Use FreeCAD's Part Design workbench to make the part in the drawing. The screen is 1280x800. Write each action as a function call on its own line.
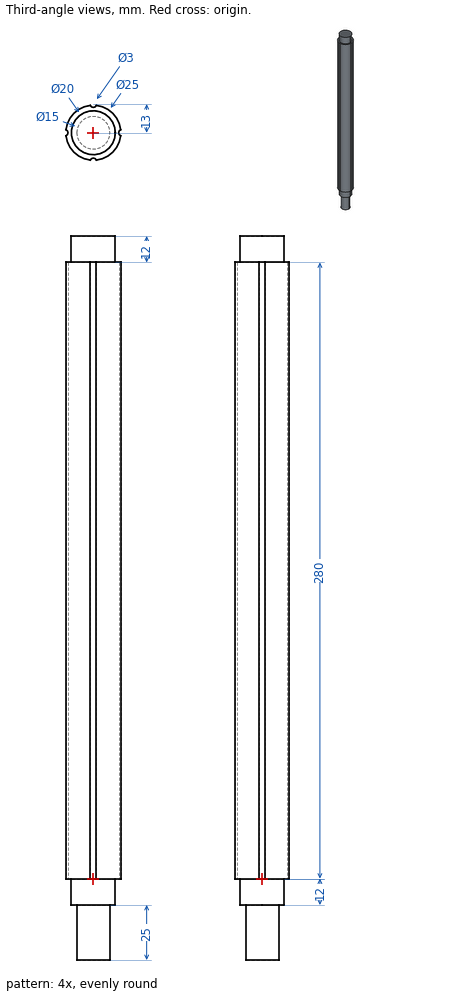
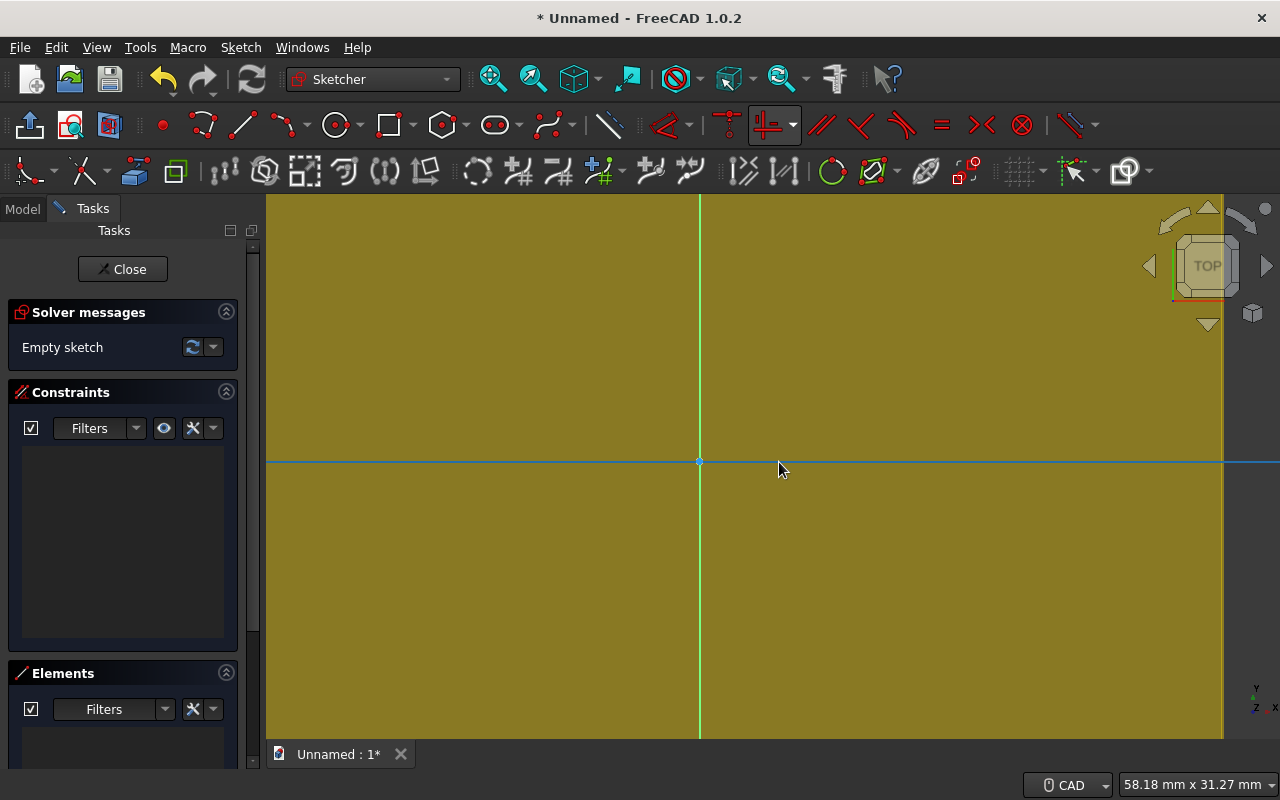
click(336, 126)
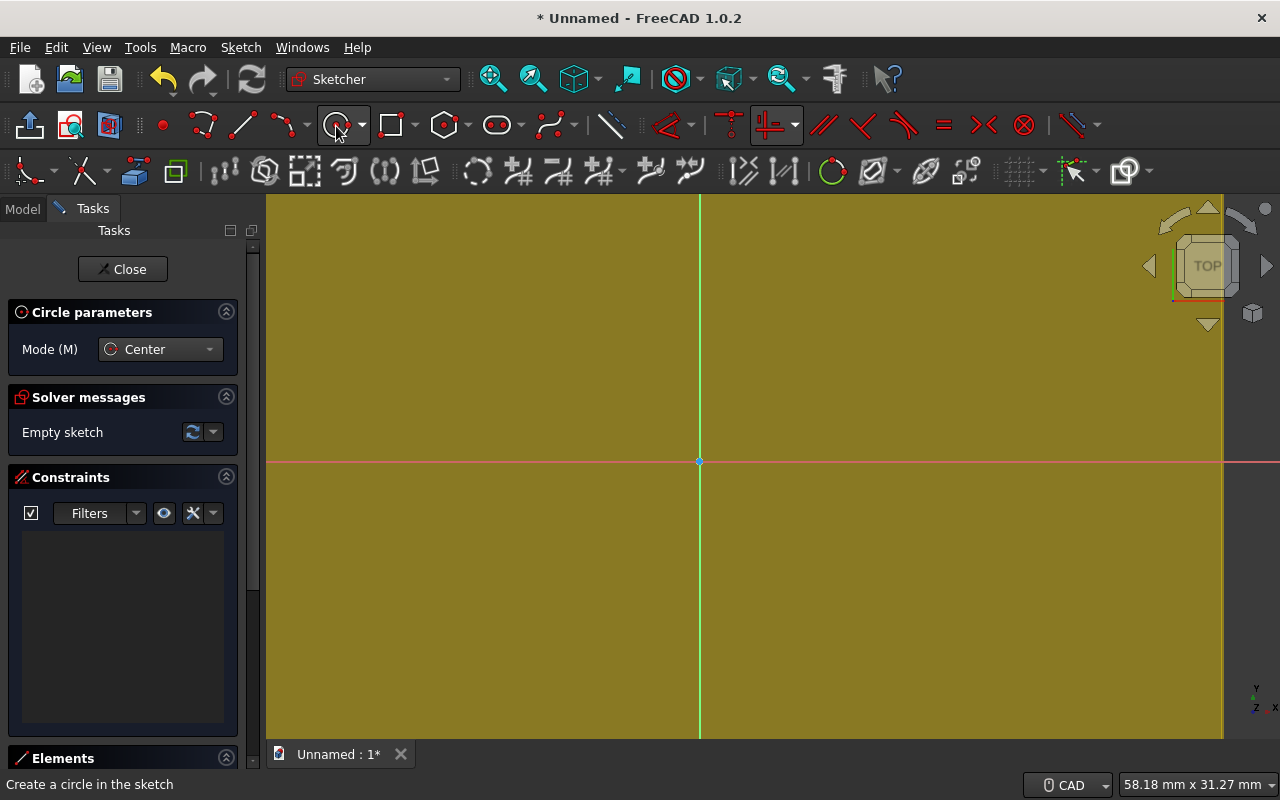
click(700, 462)
click(823, 339)
key(Escape)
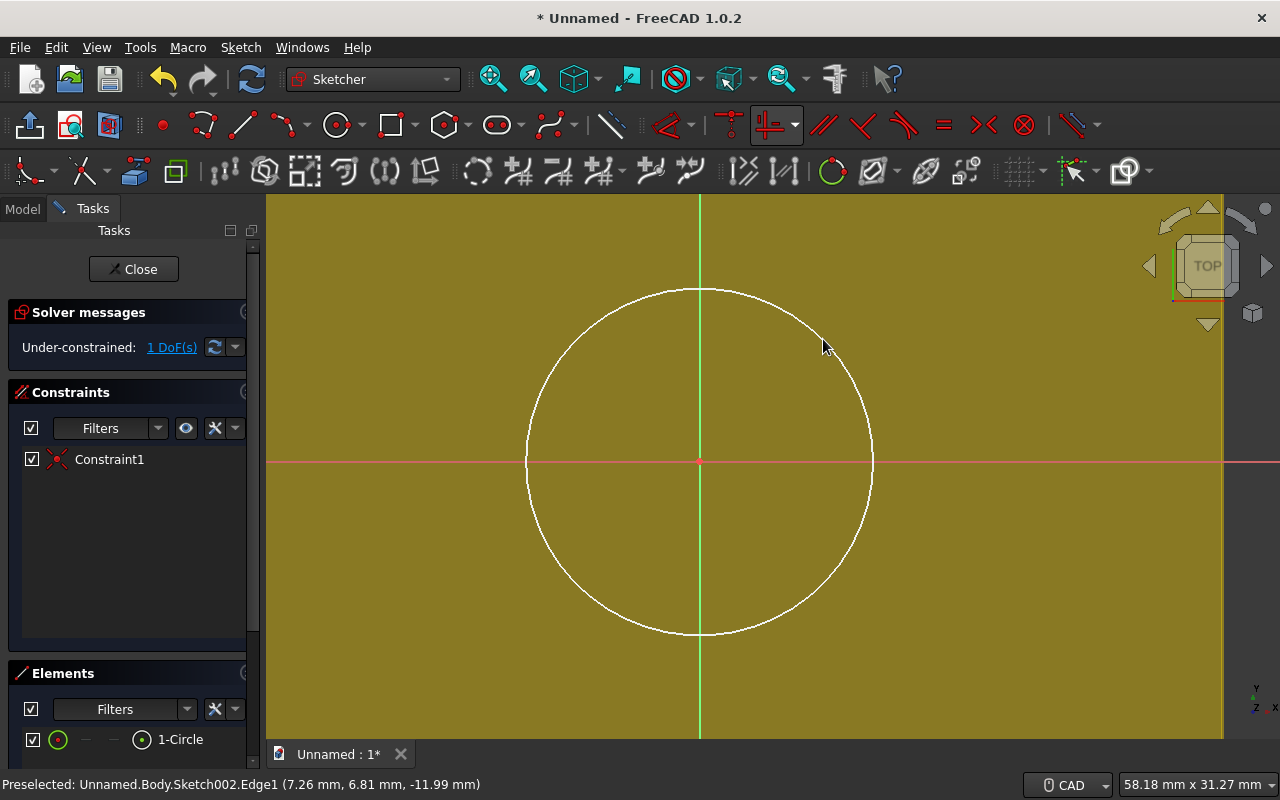
key(d)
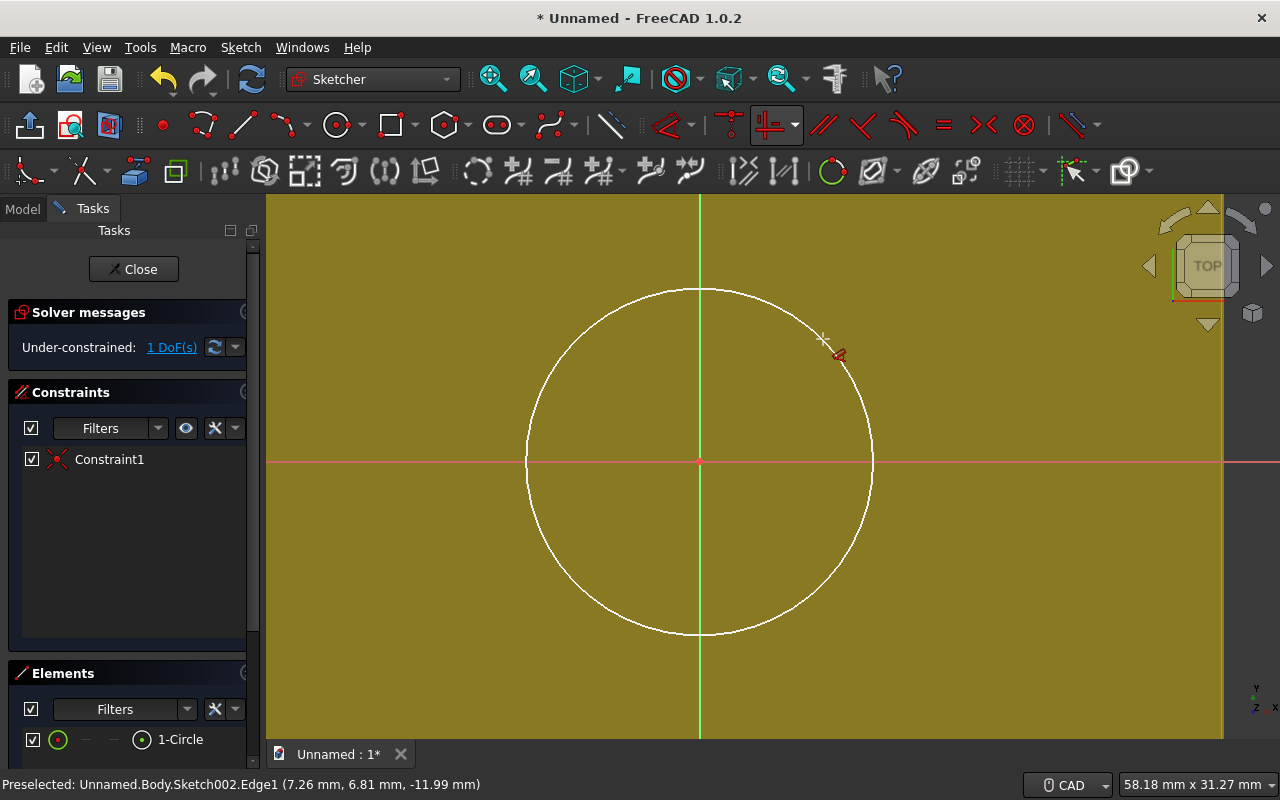
click(822, 339)
click(845, 316)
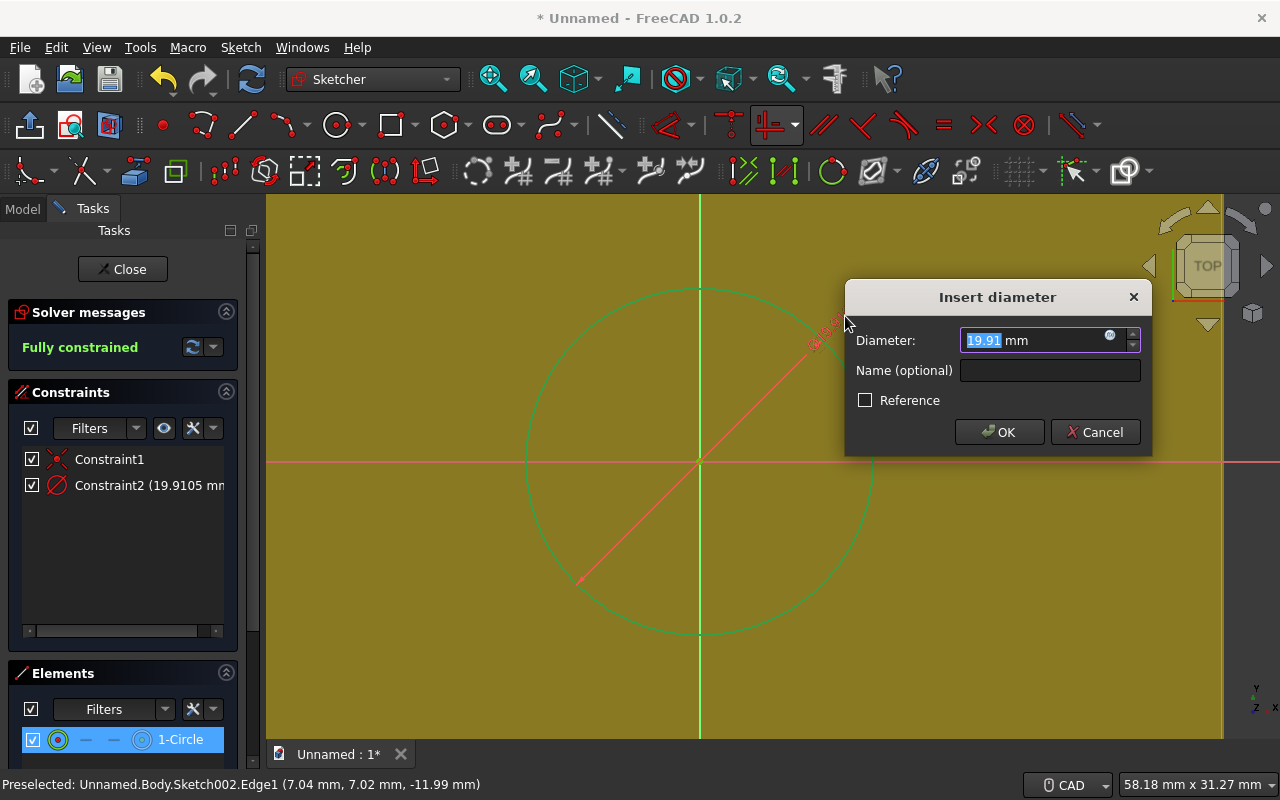
text(20)
key(Return)
key(Escape)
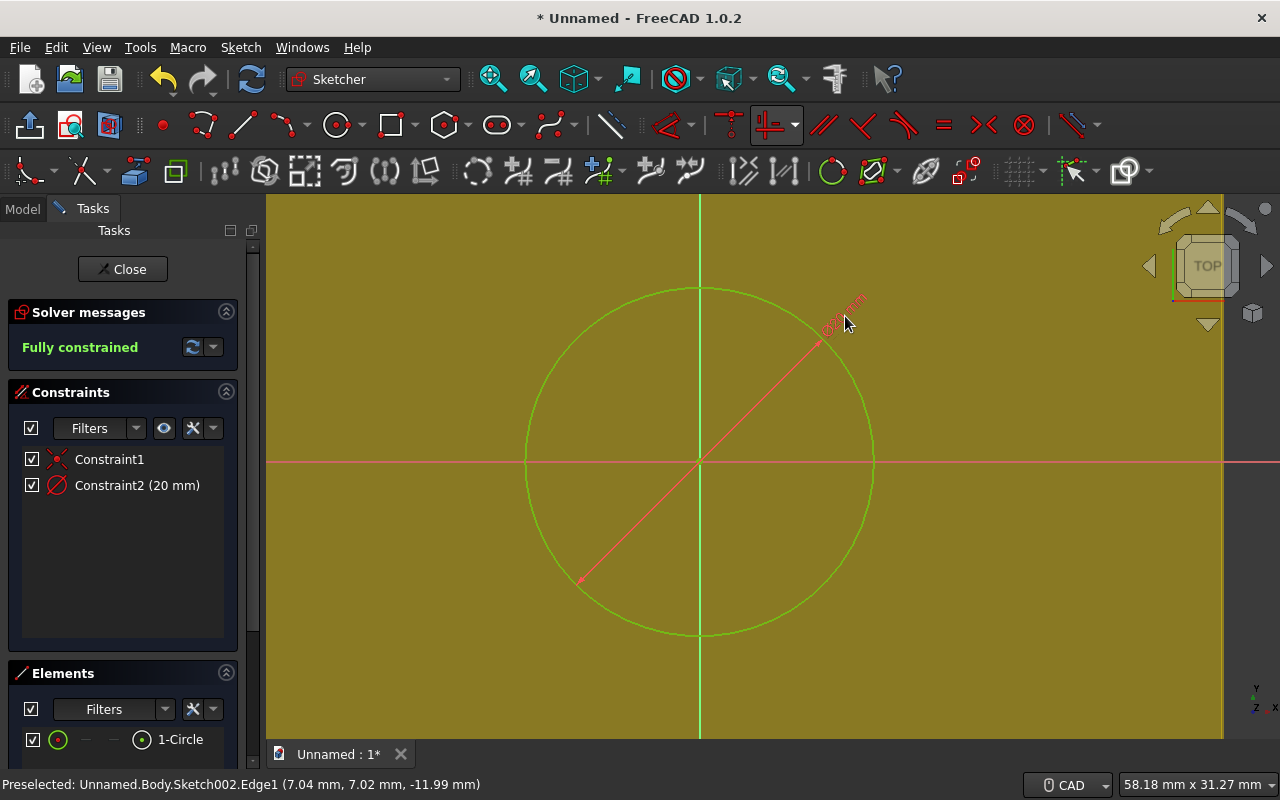
click(123, 269)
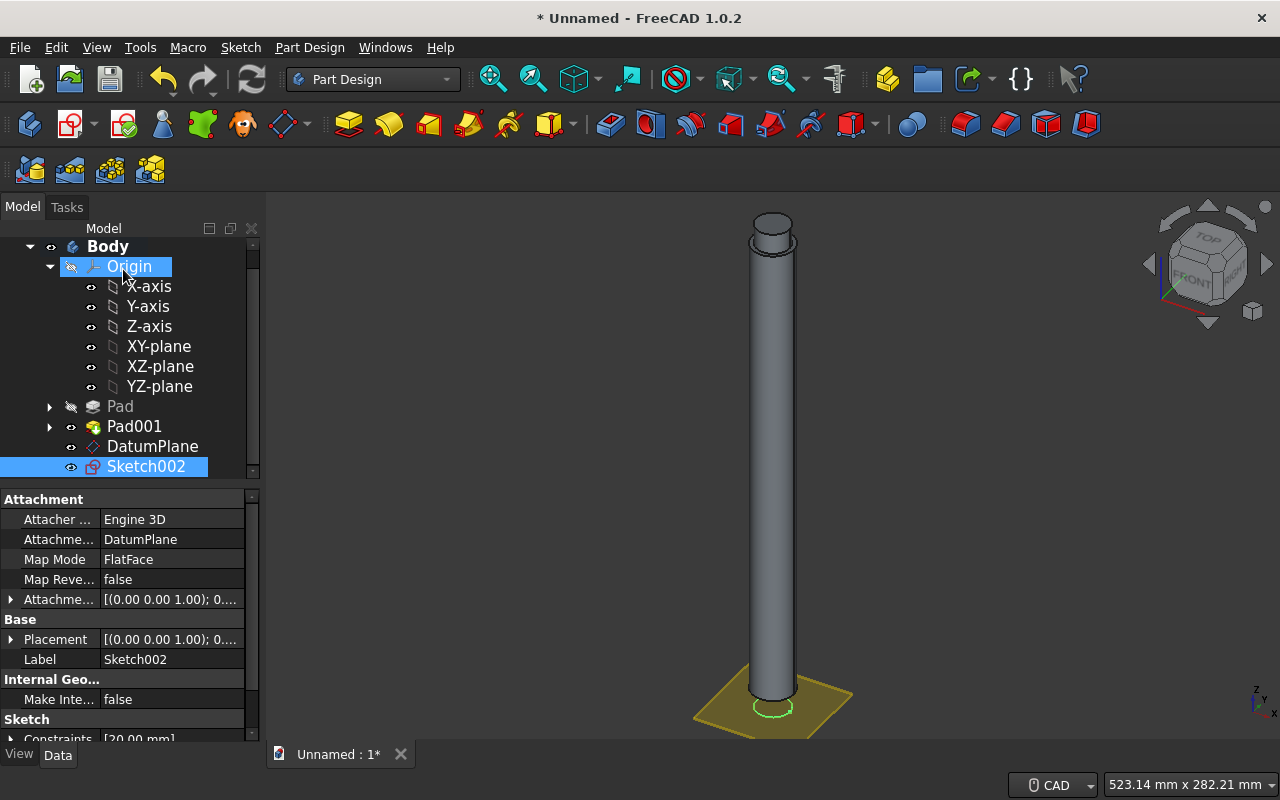
click(350, 124)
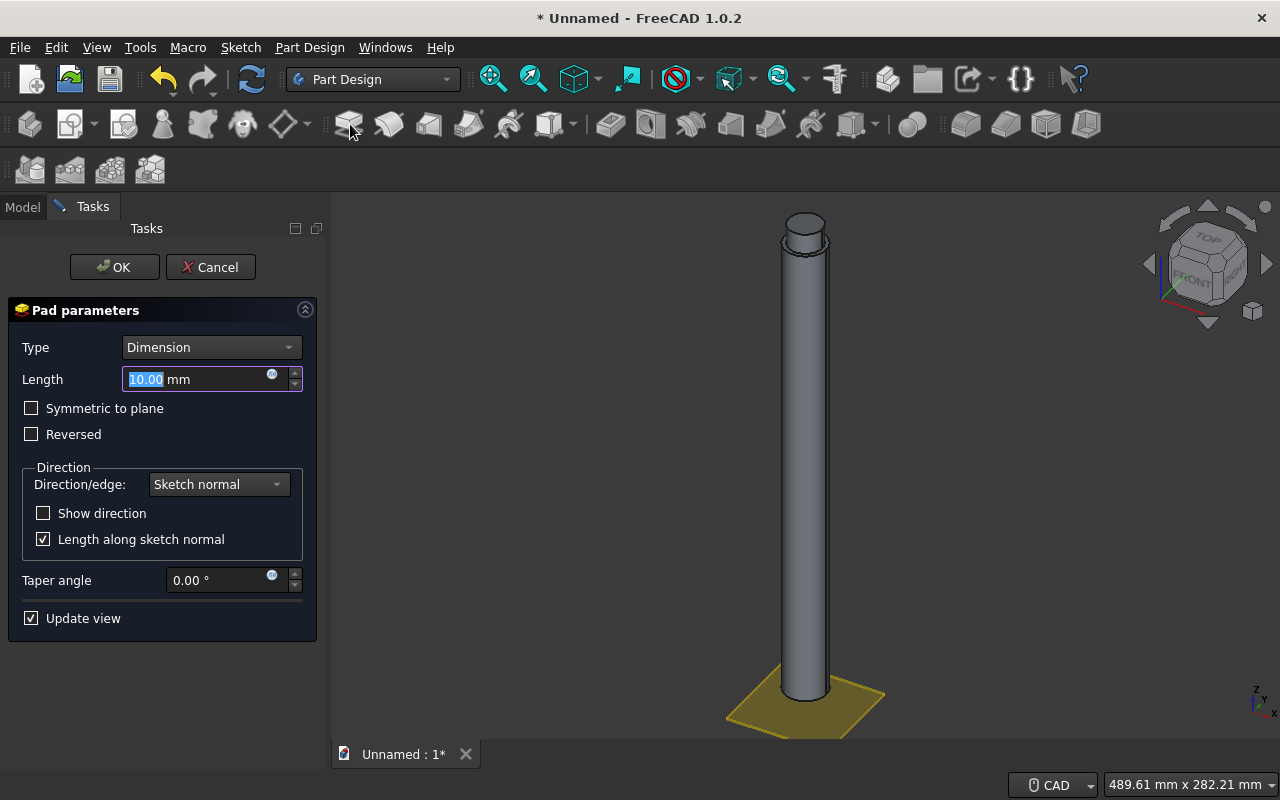
text(12)
key(Tab)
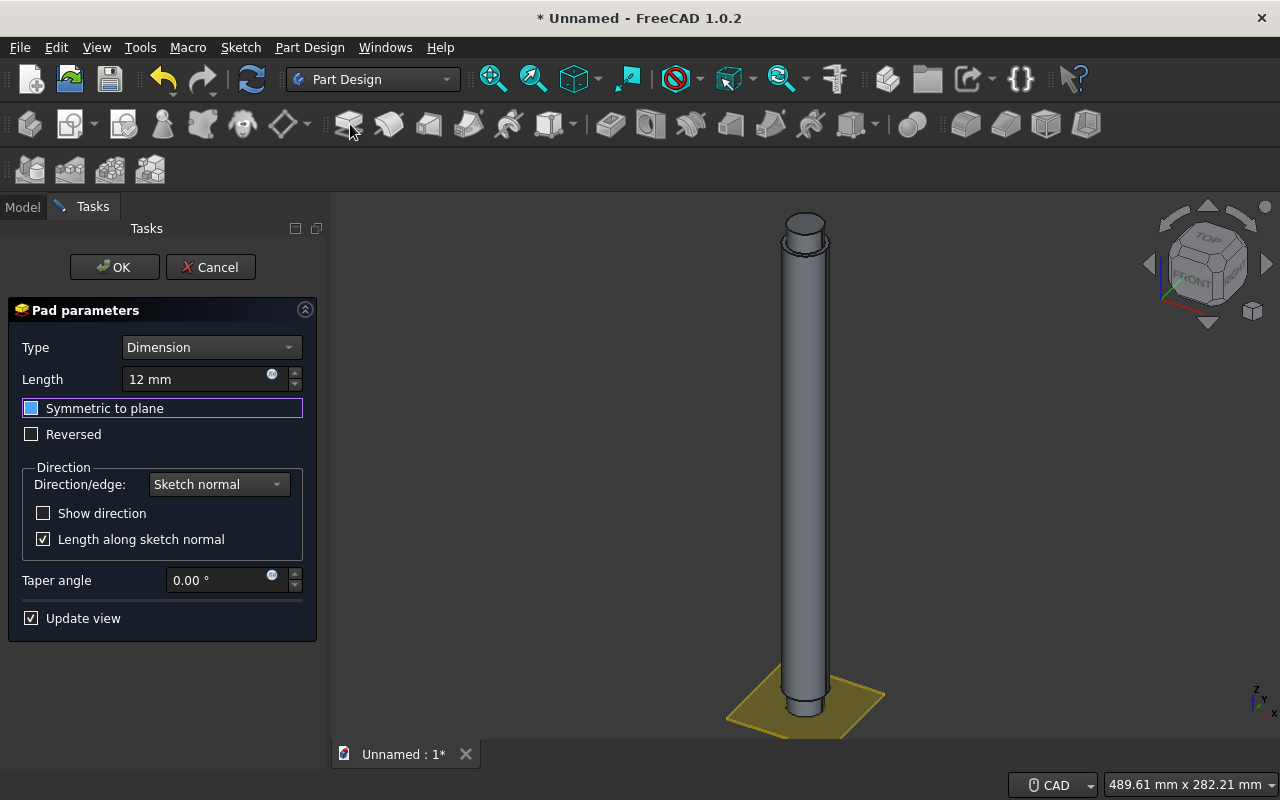
click(115, 267)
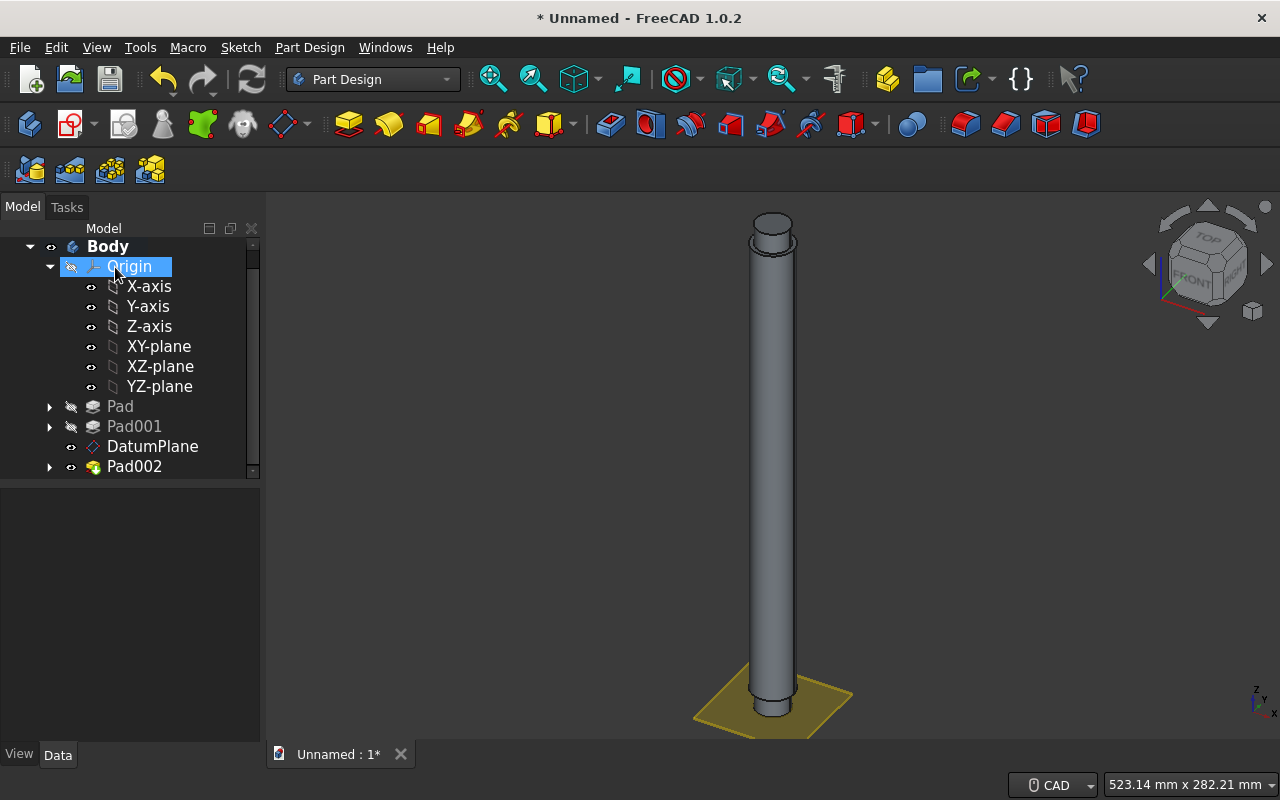
click(116, 447)
key(space)